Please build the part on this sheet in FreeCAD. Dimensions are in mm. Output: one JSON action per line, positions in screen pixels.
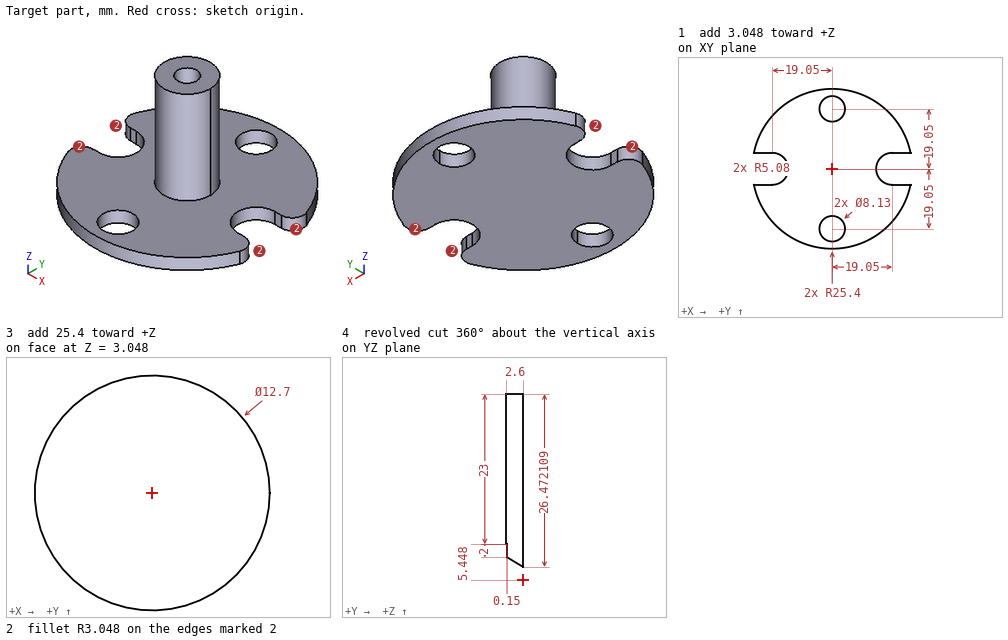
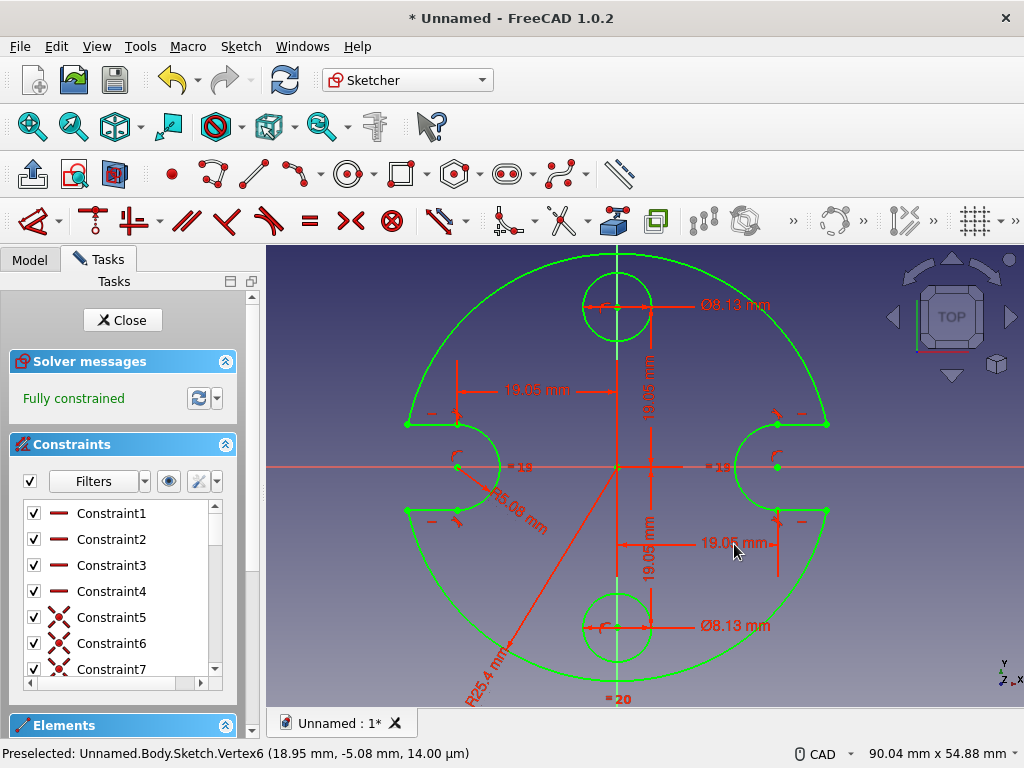
{"action": "left_click", "coordinate": [123, 320]}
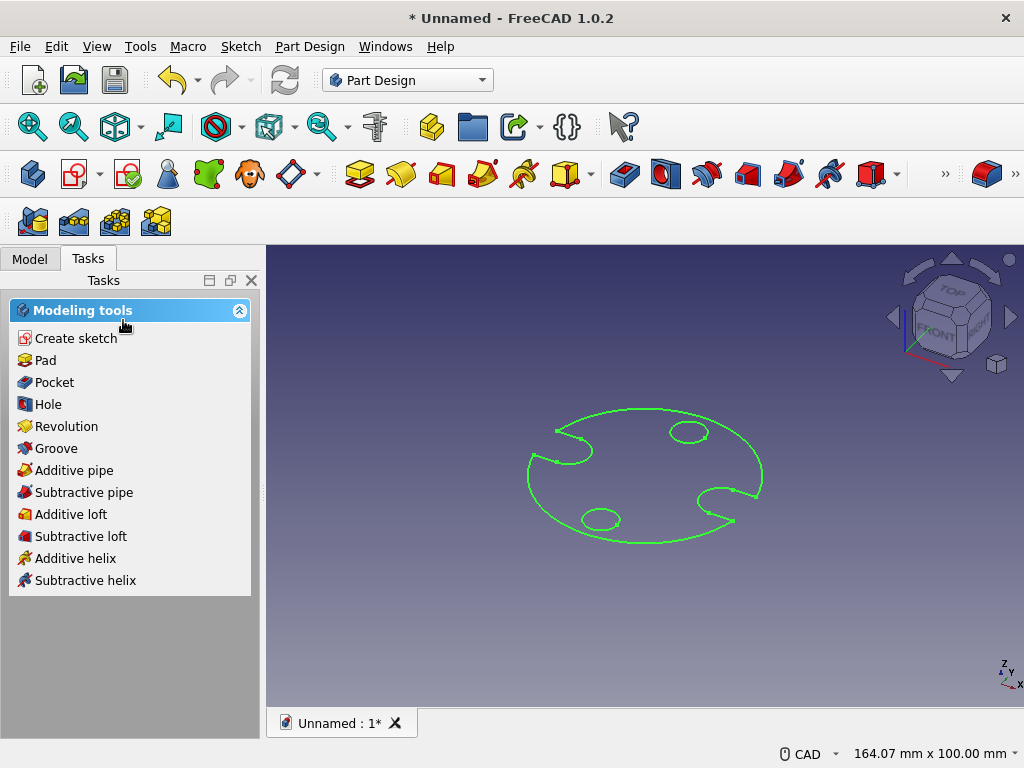
{"action": "left_click", "coordinate": [360, 174]}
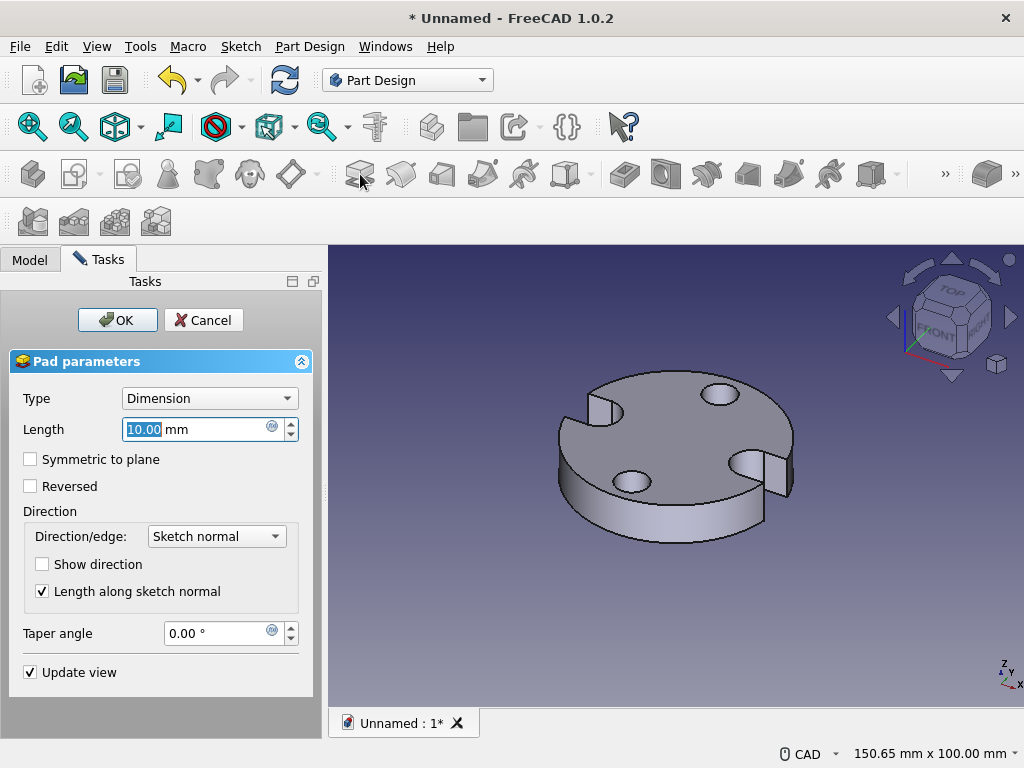
{"action": "type", "text": "3.048"}
{"action": "key", "text": "Tab"}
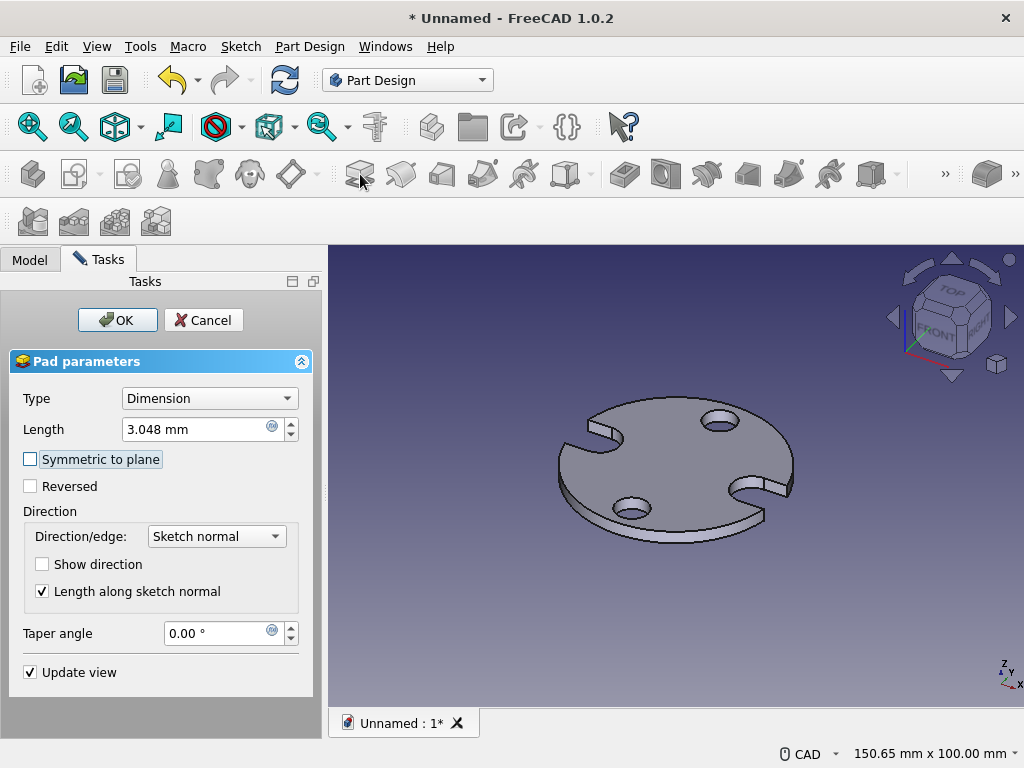
{"action": "left_click", "coordinate": [118, 320]}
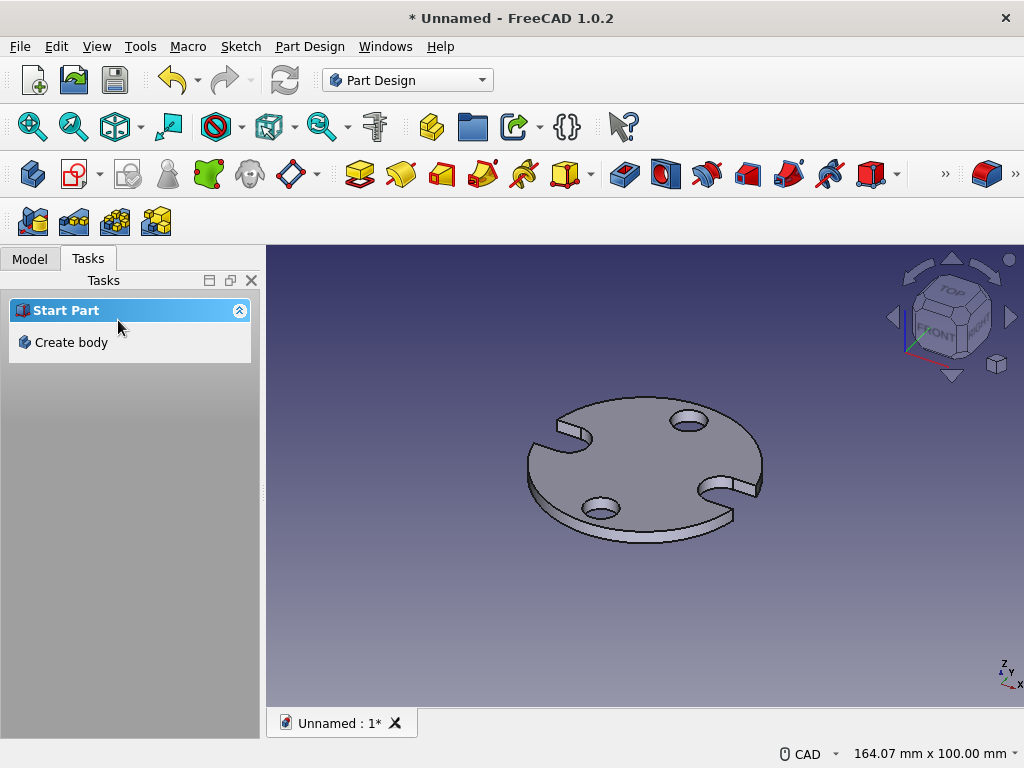
{"action": "left_click", "coordinate": [33, 128]}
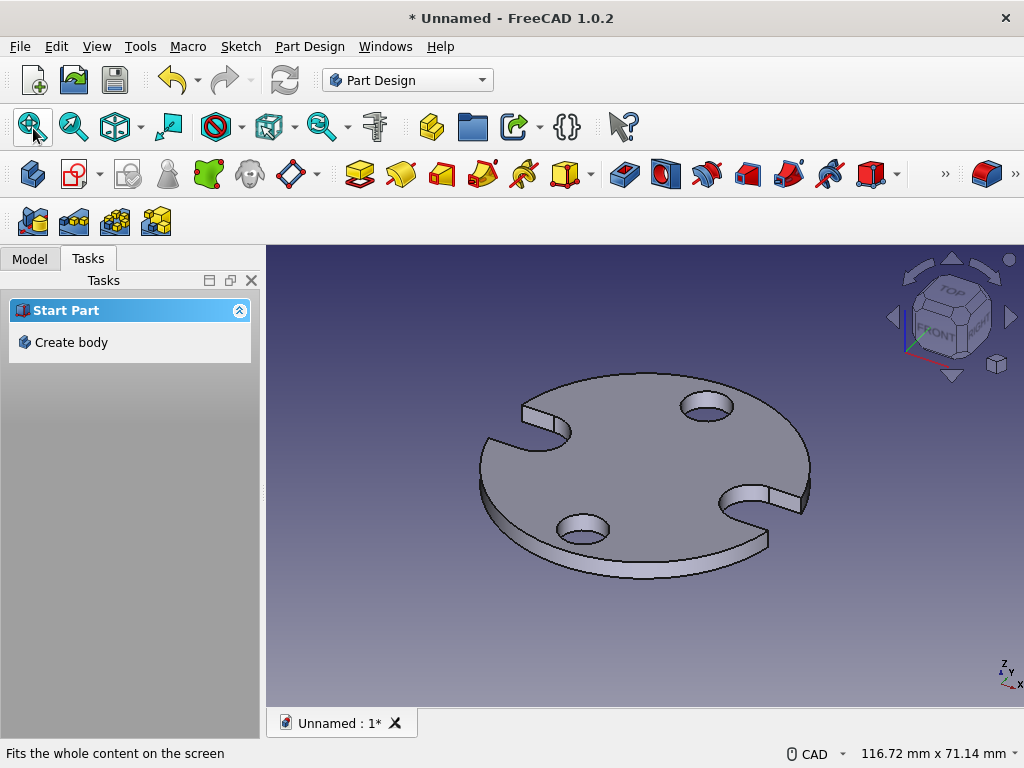
{"action": "left_click", "coordinate": [801, 505]}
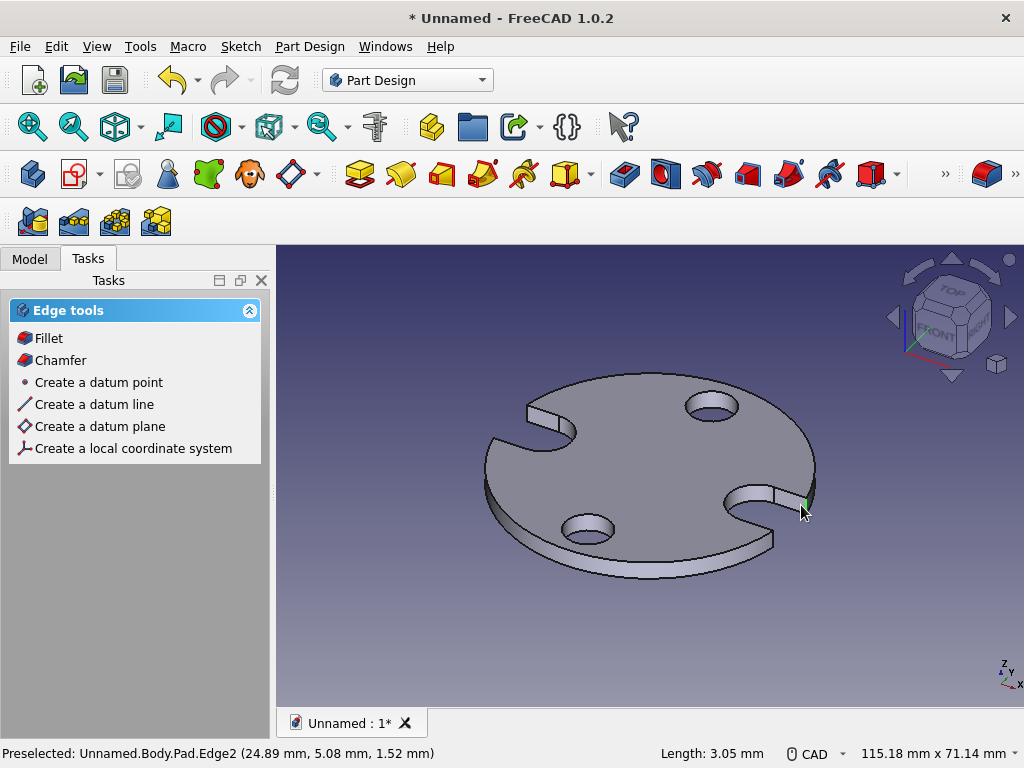
{"action": "scroll", "coordinate": [527, 412], "scroll_direction": "up", "scroll_amount": 4}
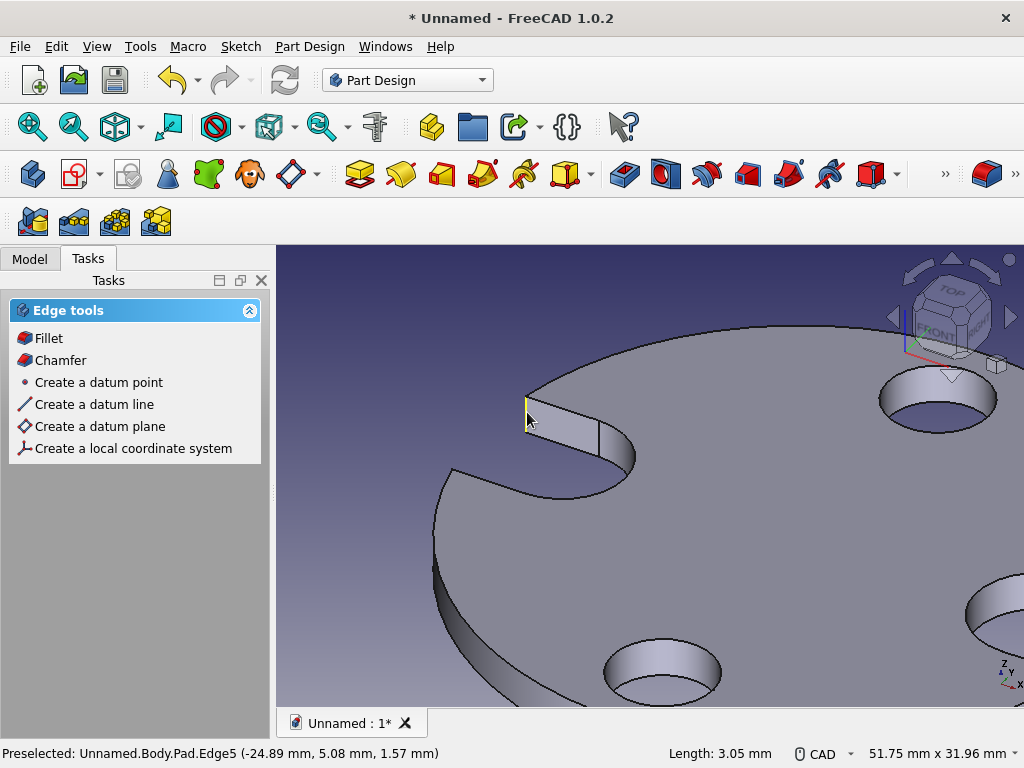
{"action": "left_click", "coordinate": [33, 128]}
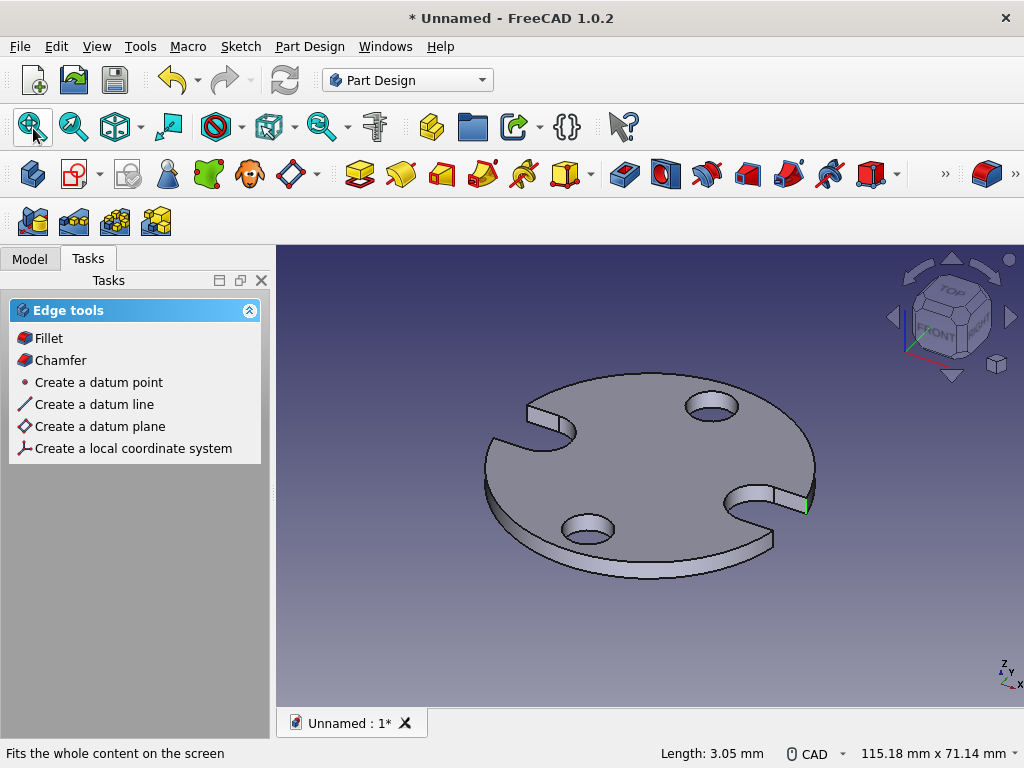
{"action": "key", "text": "0"}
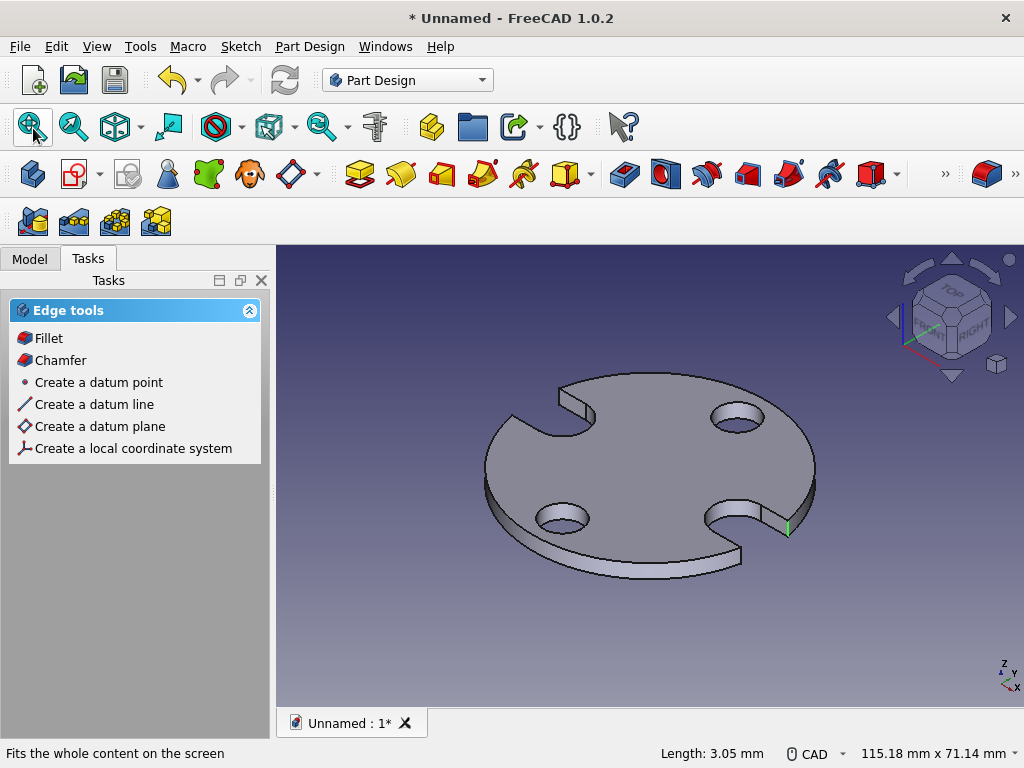
{"action": "scroll", "coordinate": [559, 396], "scroll_direction": "up", "scroll_amount": 4}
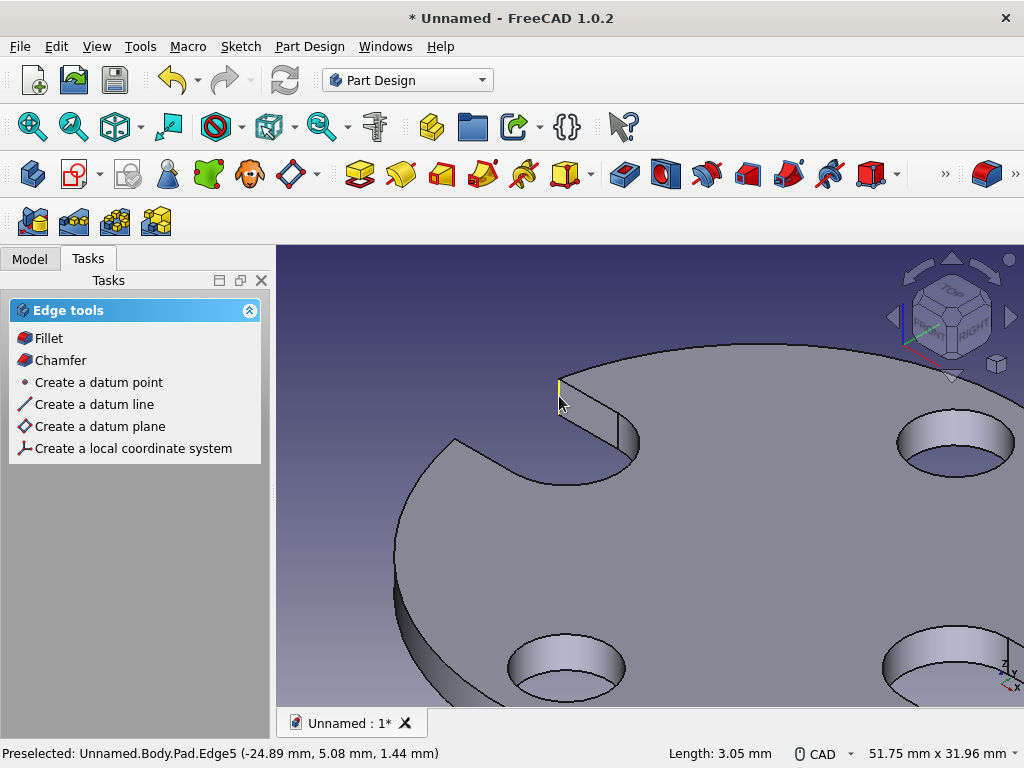
{"action": "left_click", "coordinate": [33, 128]}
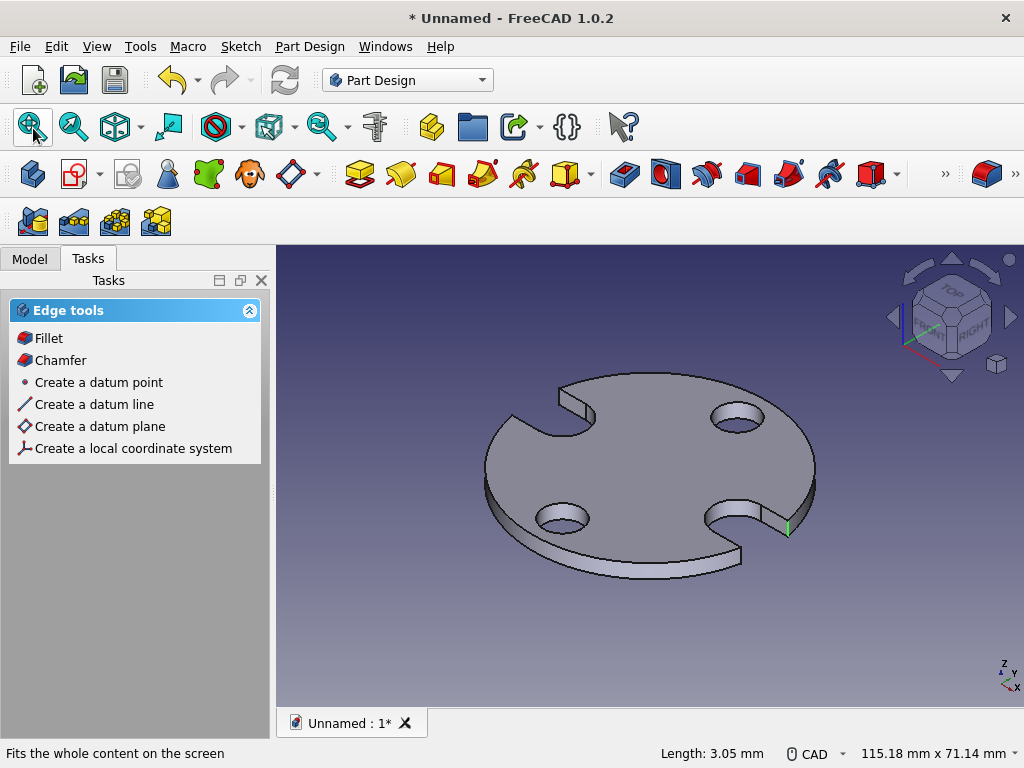
{"action": "key", "text": "2"}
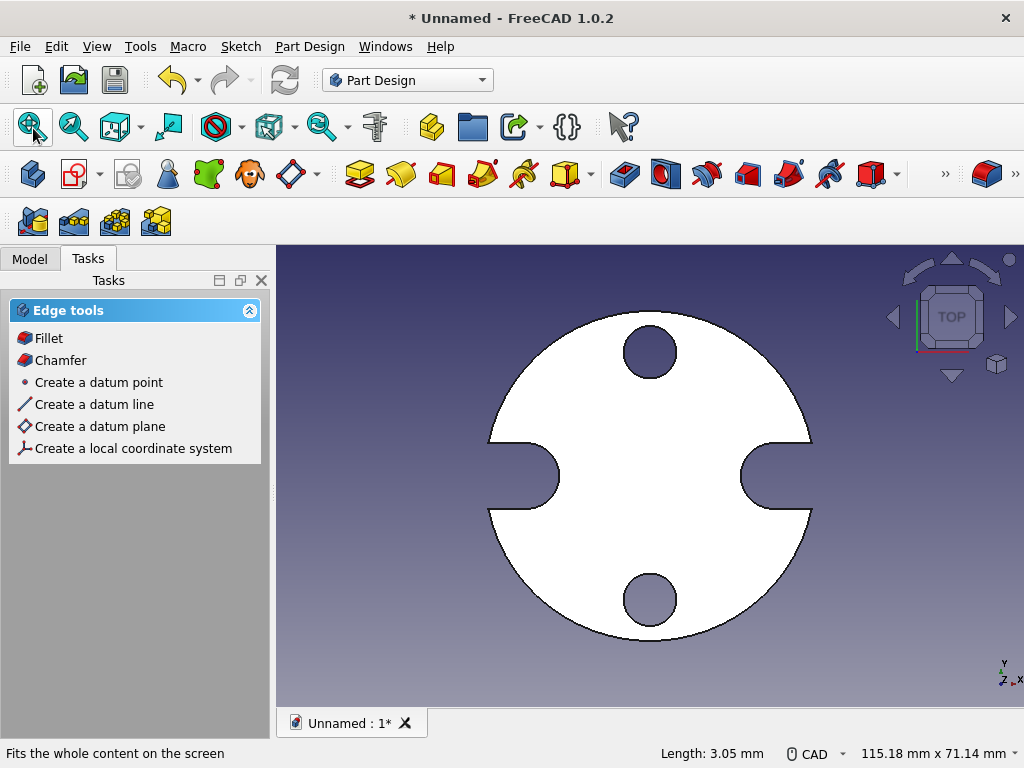
{"action": "scroll", "coordinate": [488, 442], "scroll_direction": "up", "scroll_amount": 4}